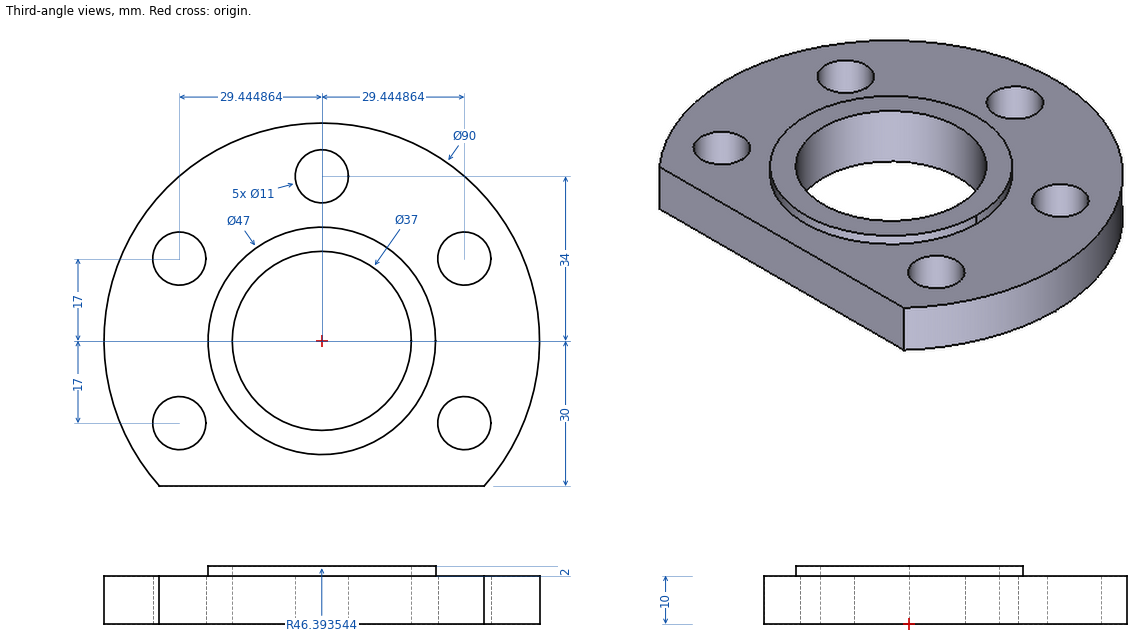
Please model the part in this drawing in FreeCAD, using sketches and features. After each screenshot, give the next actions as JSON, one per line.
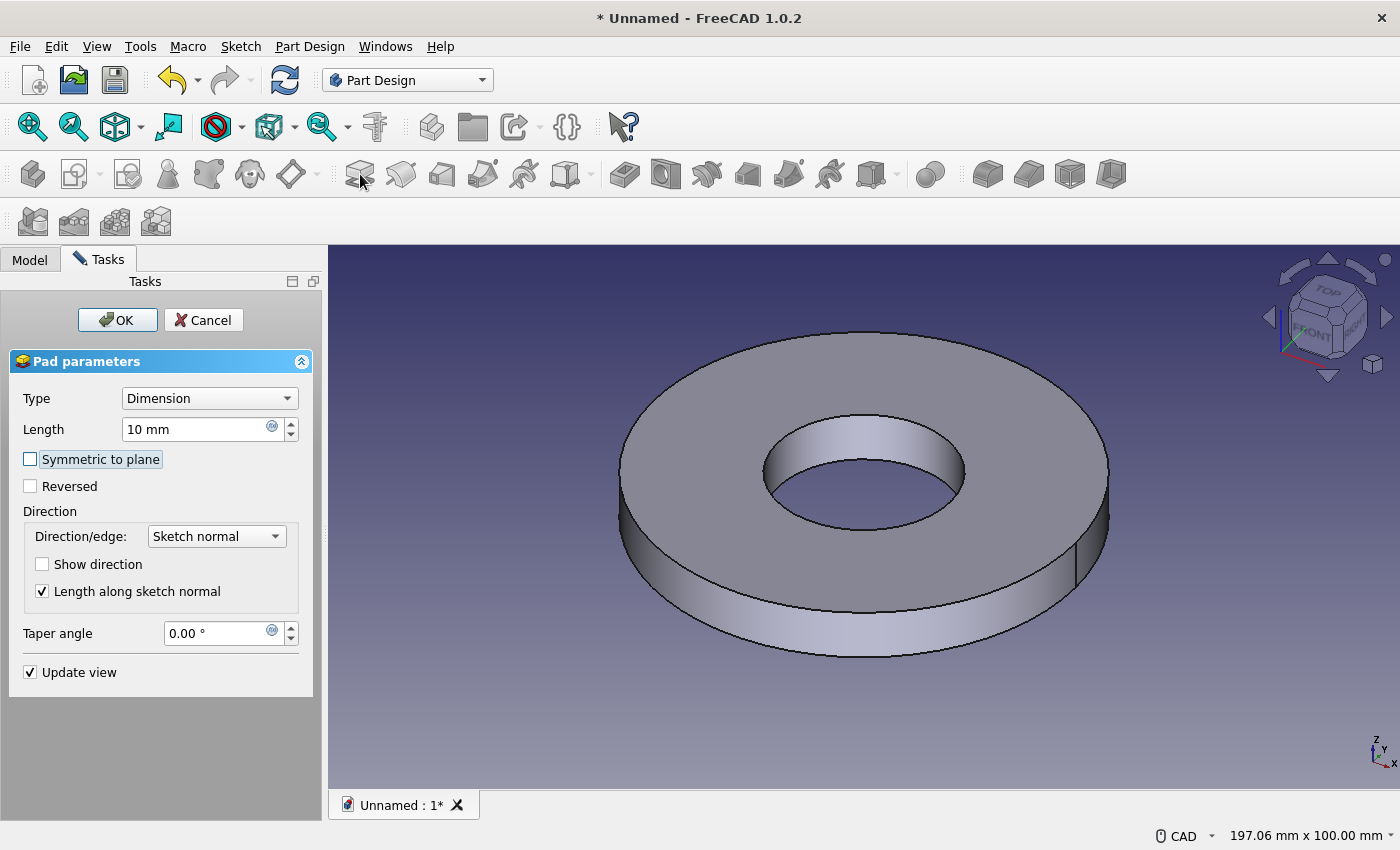
{"action": "left_click", "coordinate": [118, 320]}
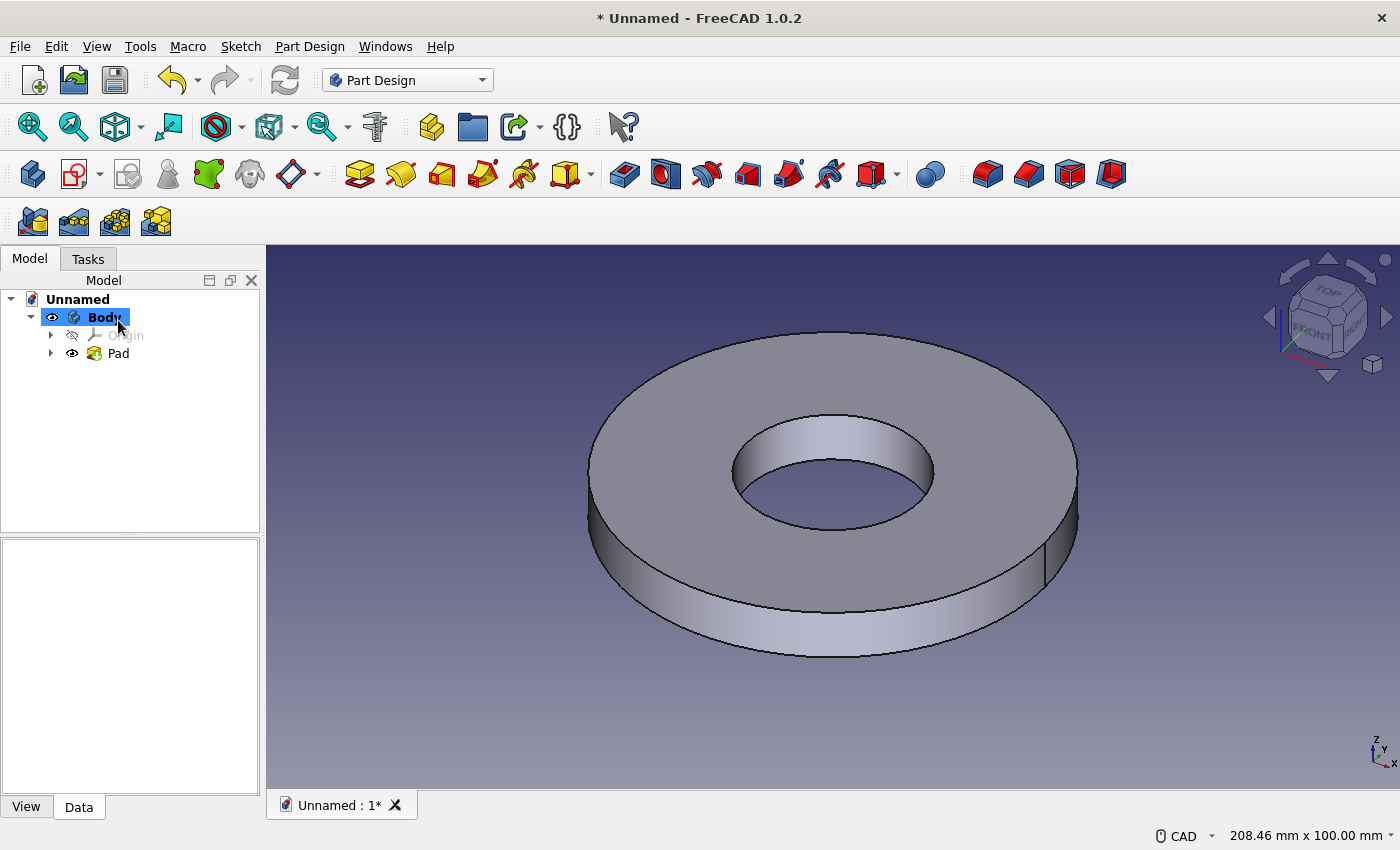
{"action": "left_click", "coordinate": [702, 521]}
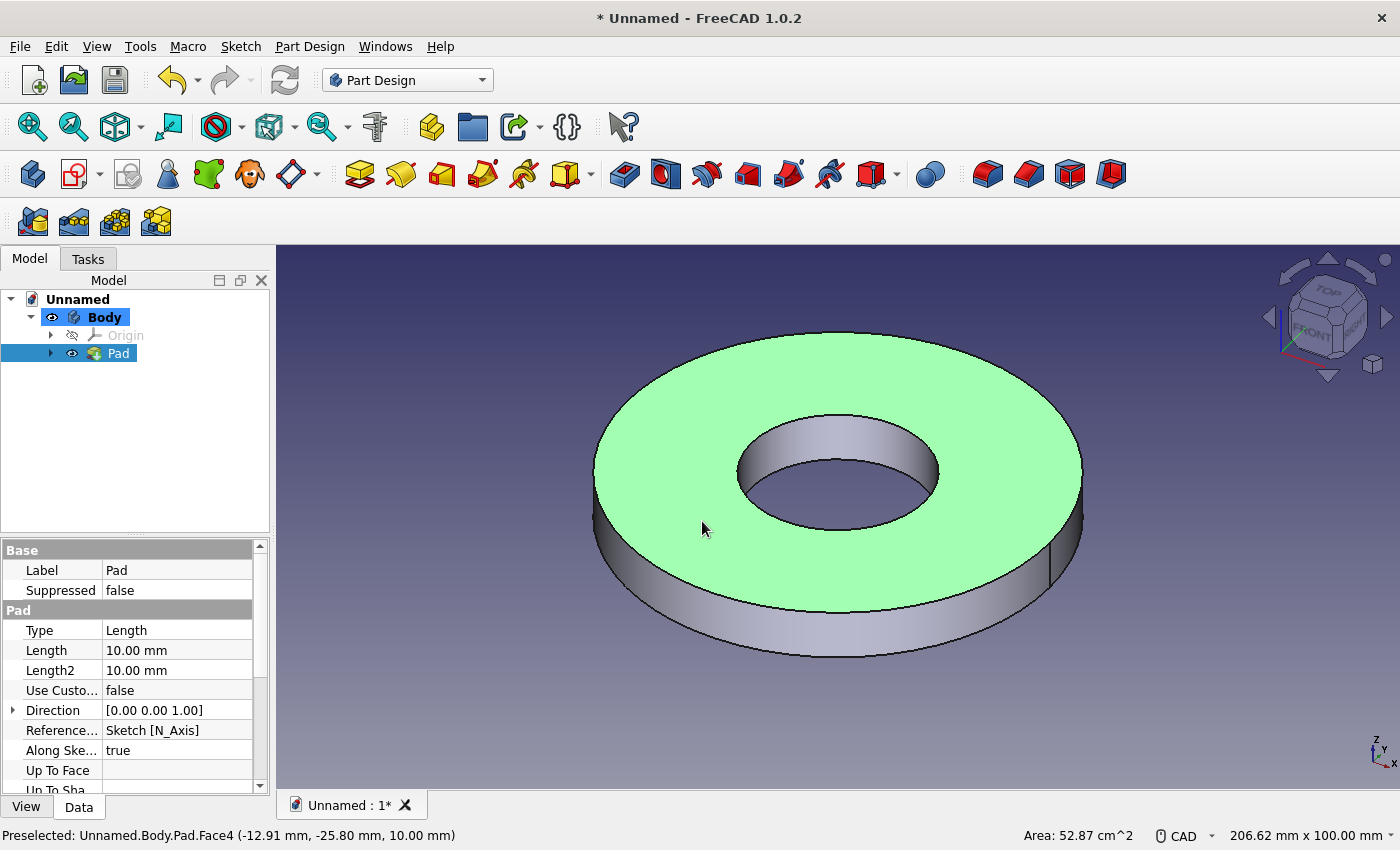
{"action": "left_click", "coordinate": [74, 174]}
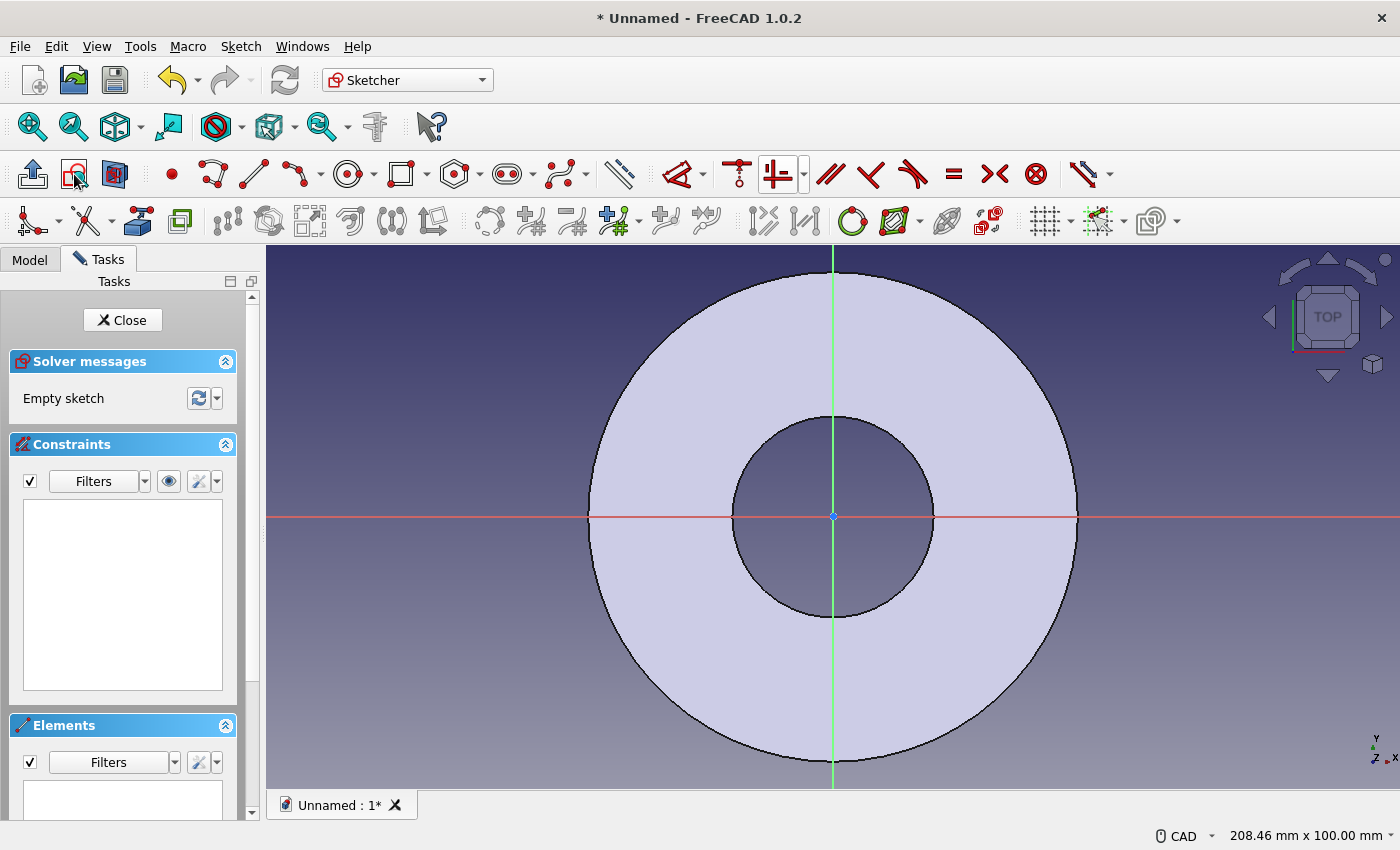
{"action": "left_click", "coordinate": [348, 174]}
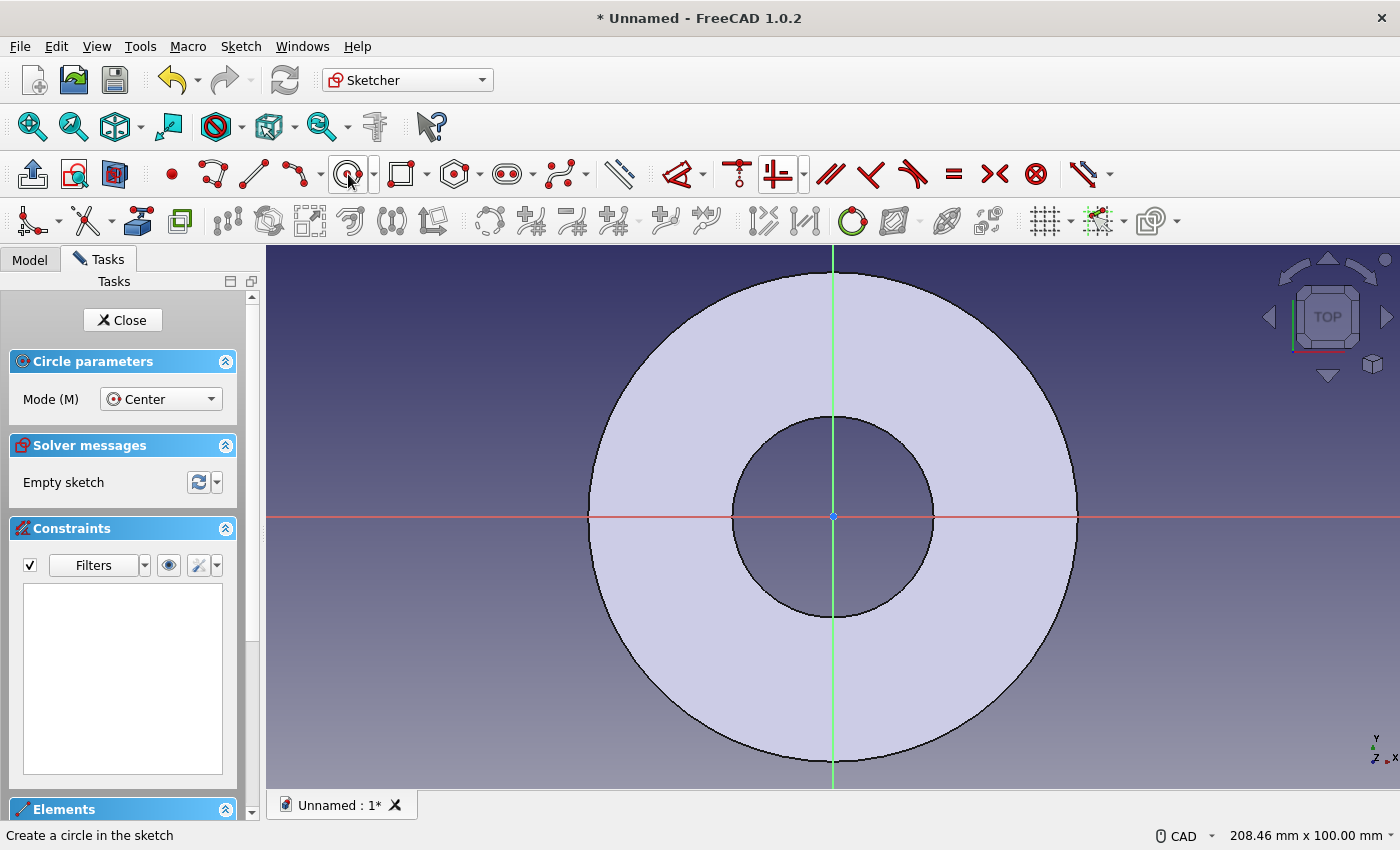
{"action": "left_click", "coordinate": [833, 517]}
{"action": "left_click", "coordinate": [923, 427]}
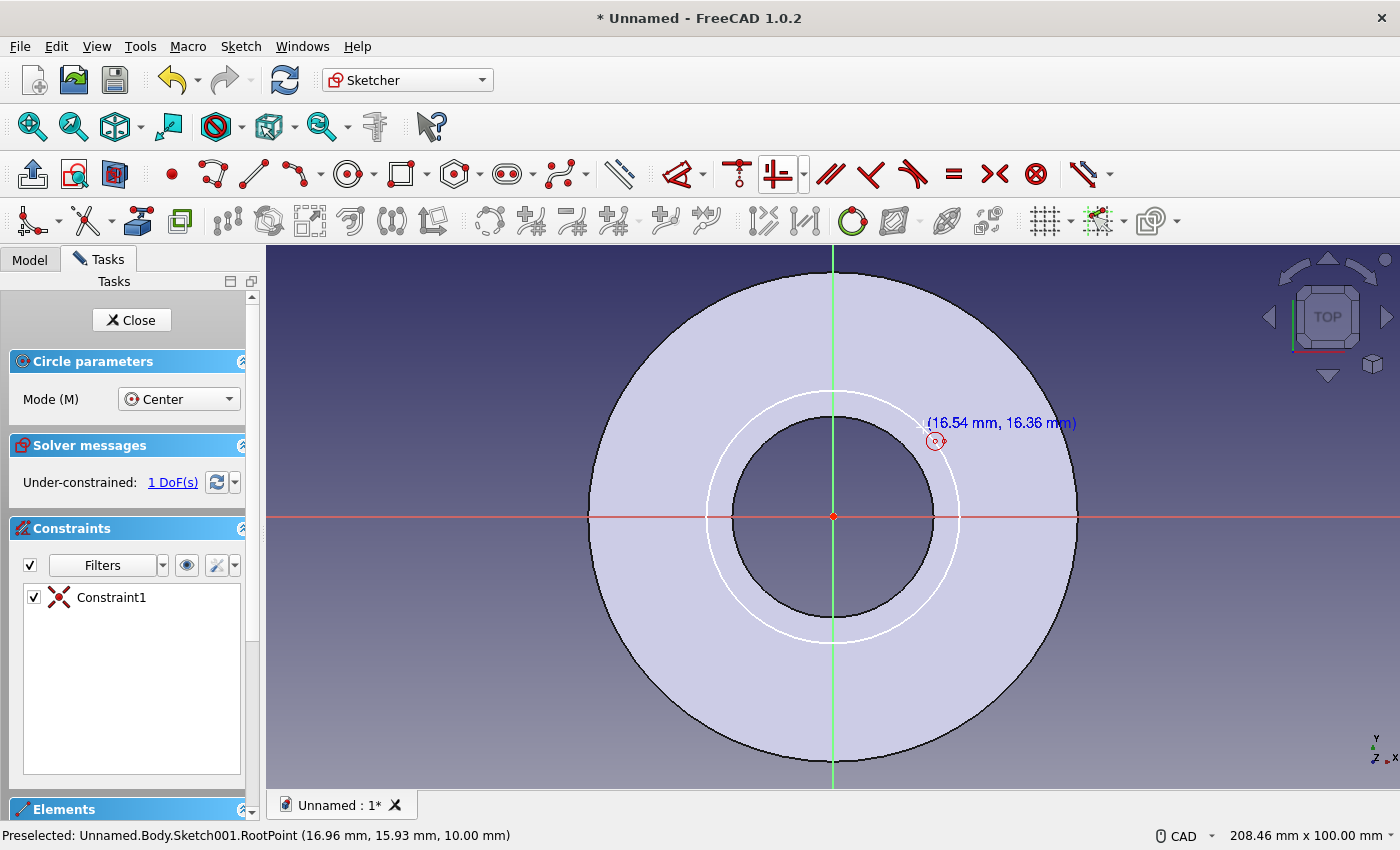
{"action": "left_click", "coordinate": [833, 517]}
{"action": "left_click", "coordinate": [904, 446]}
{"action": "key", "text": "Escape"}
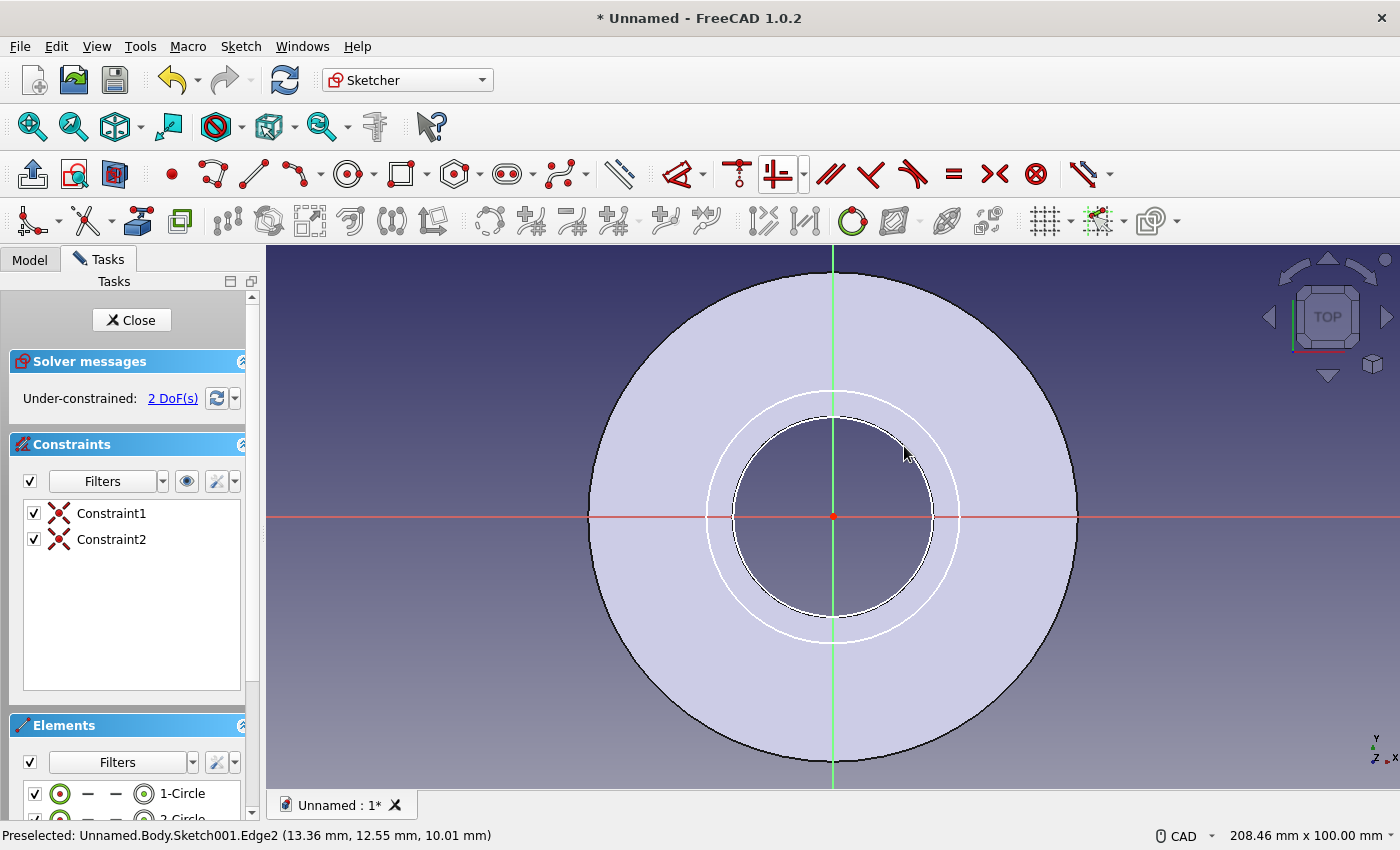
{"action": "left_click", "coordinate": [676, 174]}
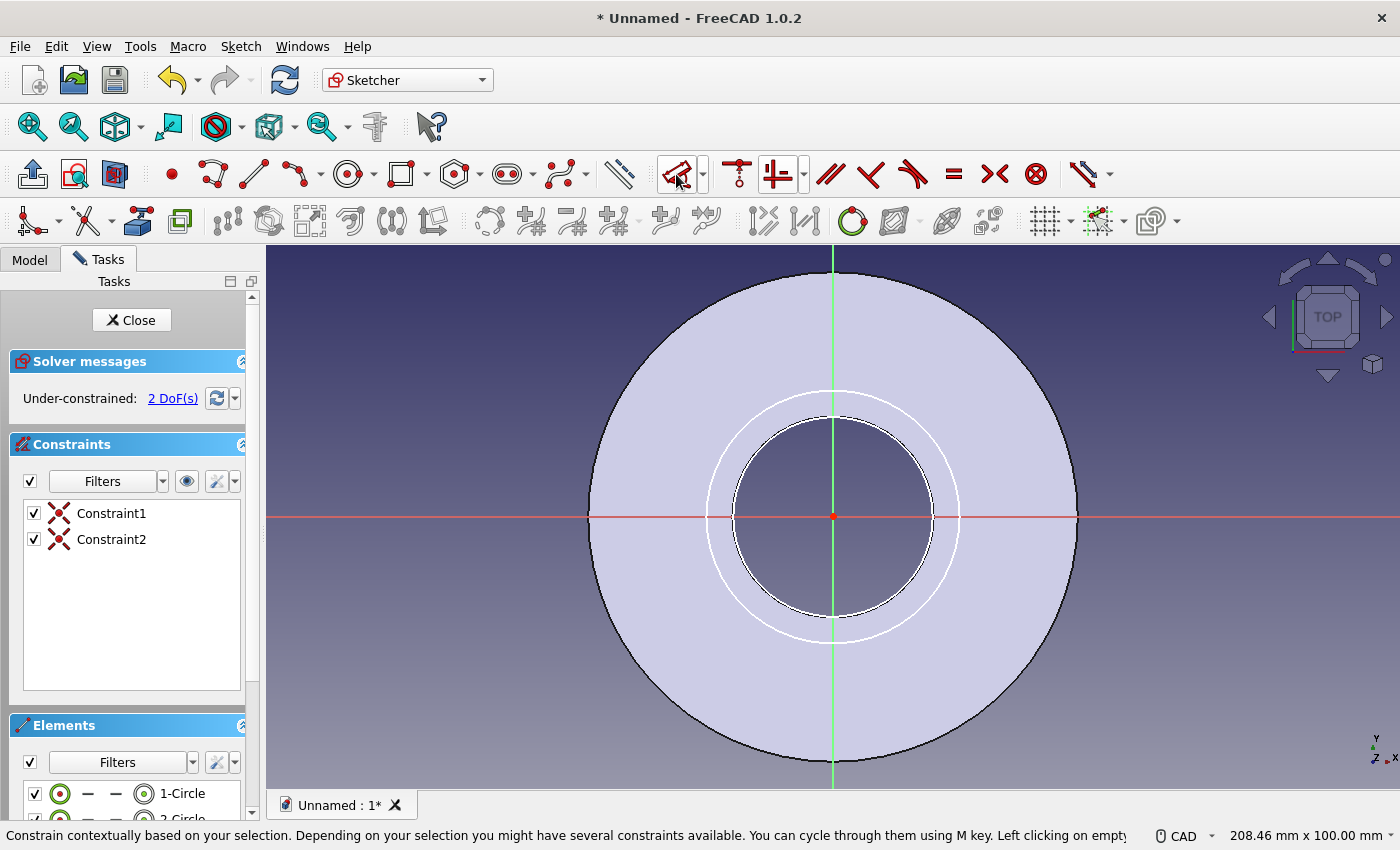
{"action": "left_click", "coordinate": [922, 427]}
{"action": "left_click", "coordinate": [945, 404]}